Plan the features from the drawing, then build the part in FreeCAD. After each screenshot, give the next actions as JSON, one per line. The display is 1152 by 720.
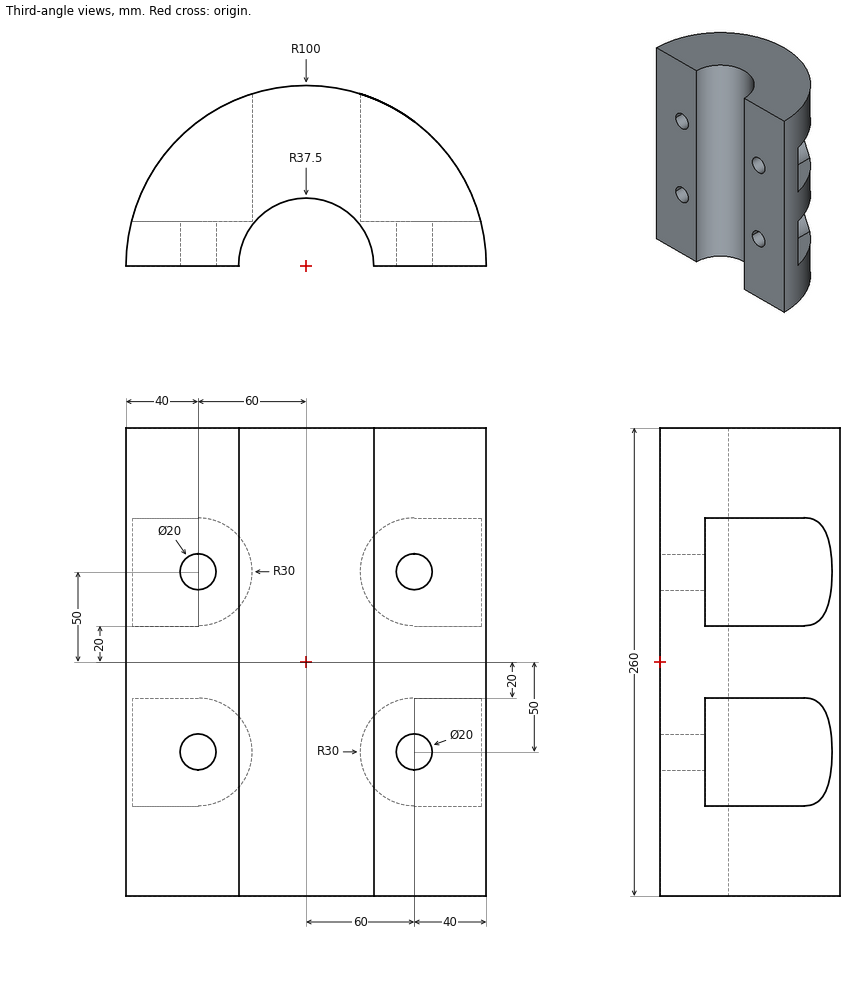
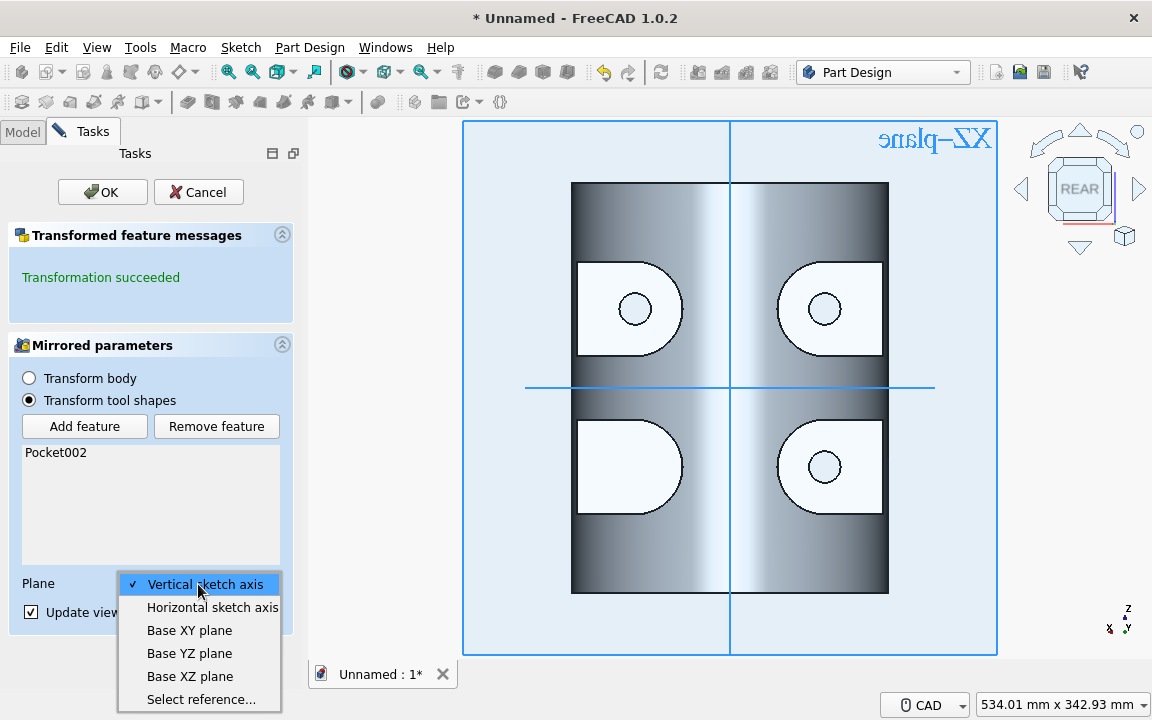
{"action": "left_click", "coordinate": [198, 654]}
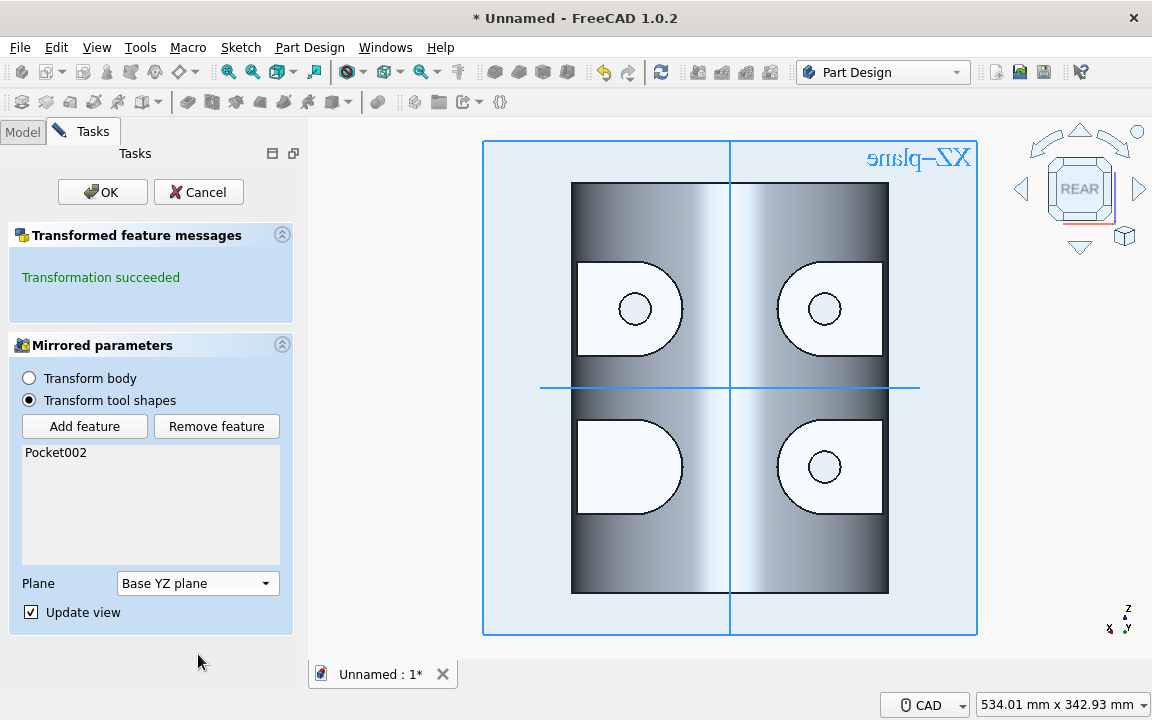
{"action": "left_click", "coordinate": [103, 192]}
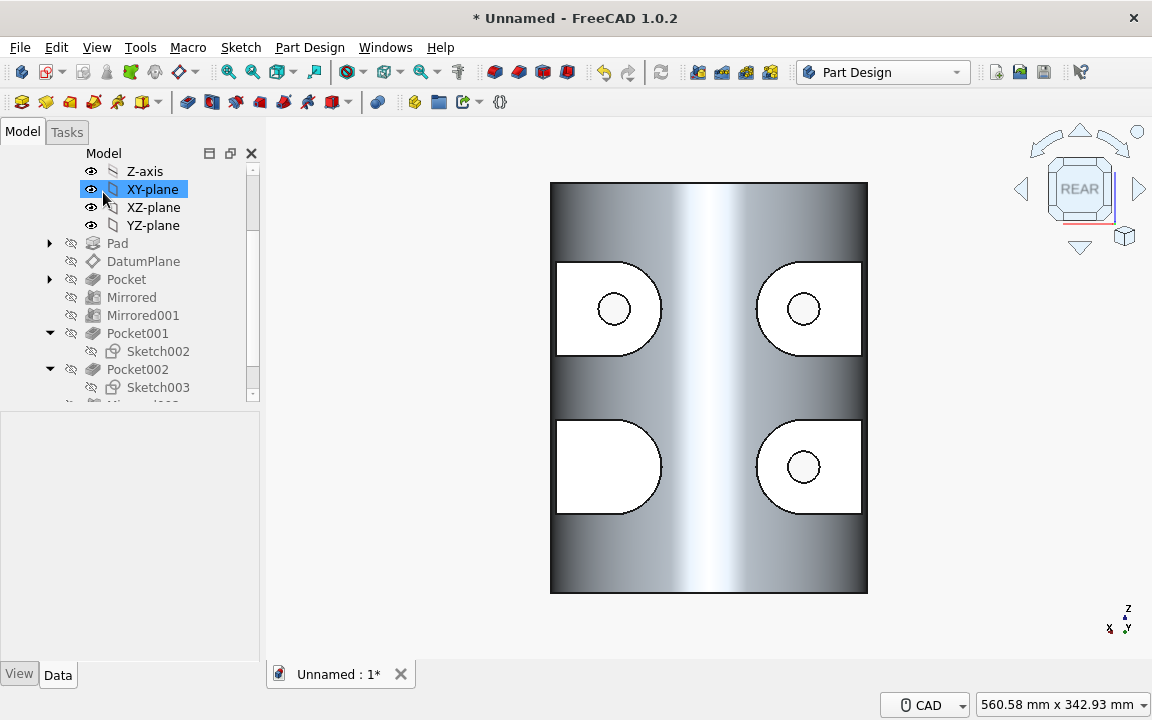
{"action": "left_click", "coordinate": [609, 466]}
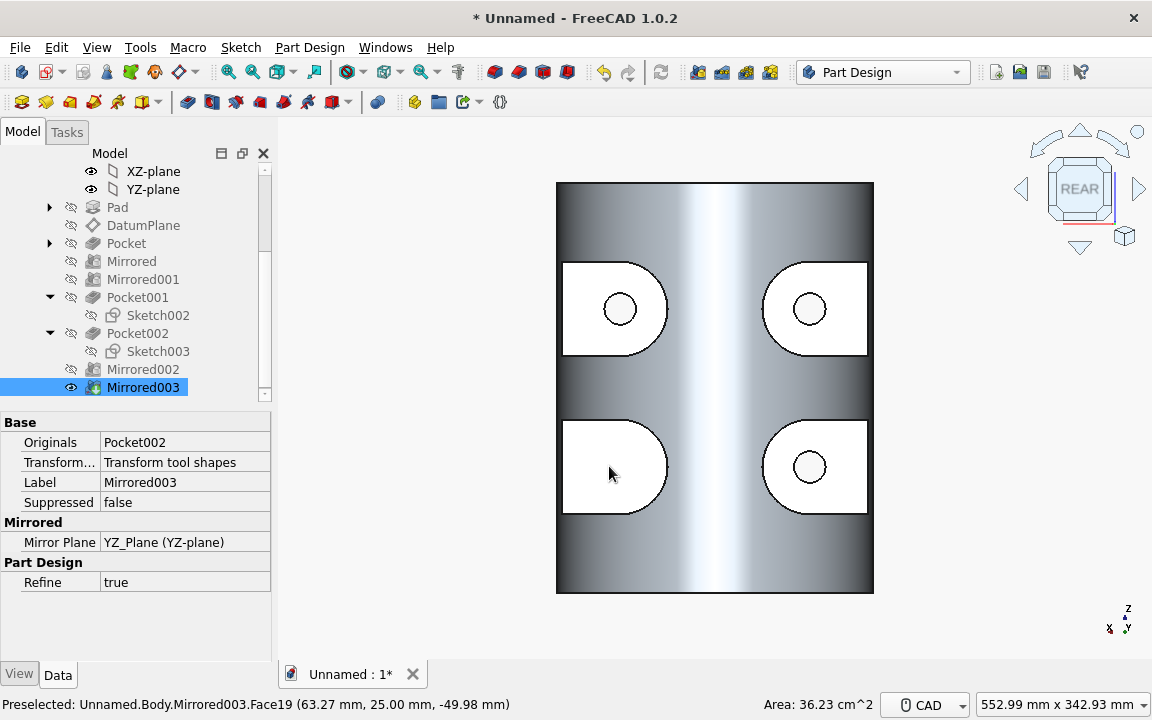
{"action": "left_click", "coordinate": [46, 72]}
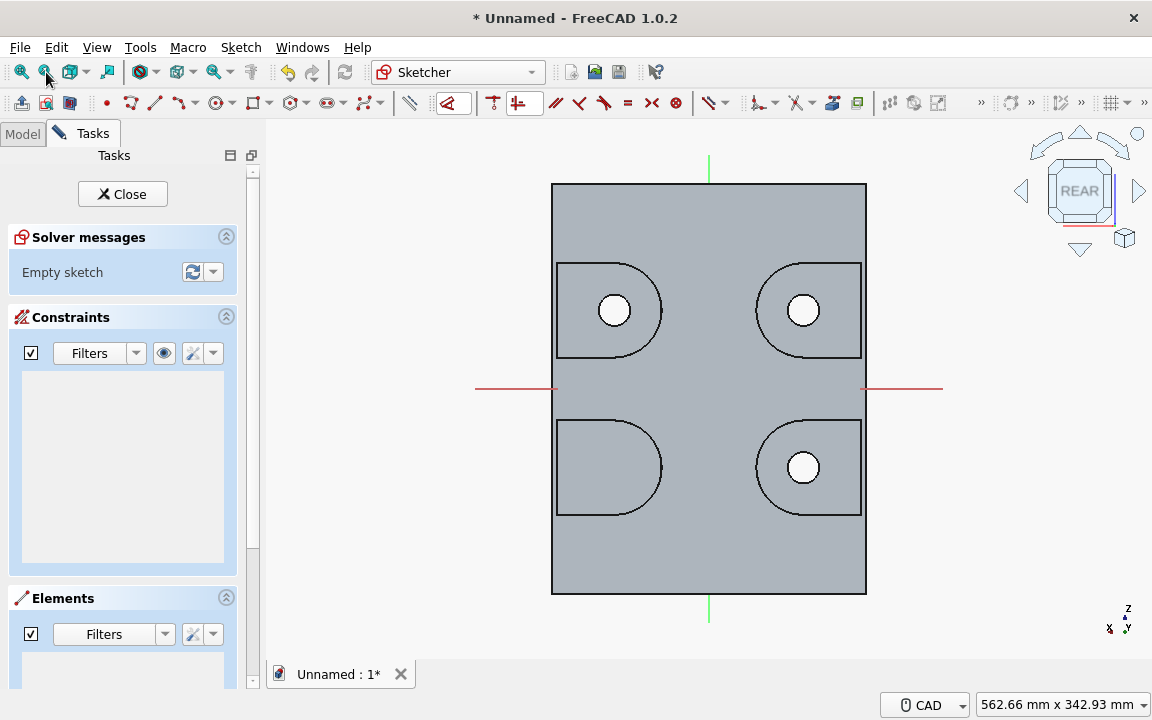
{"action": "key", "text": "q s"}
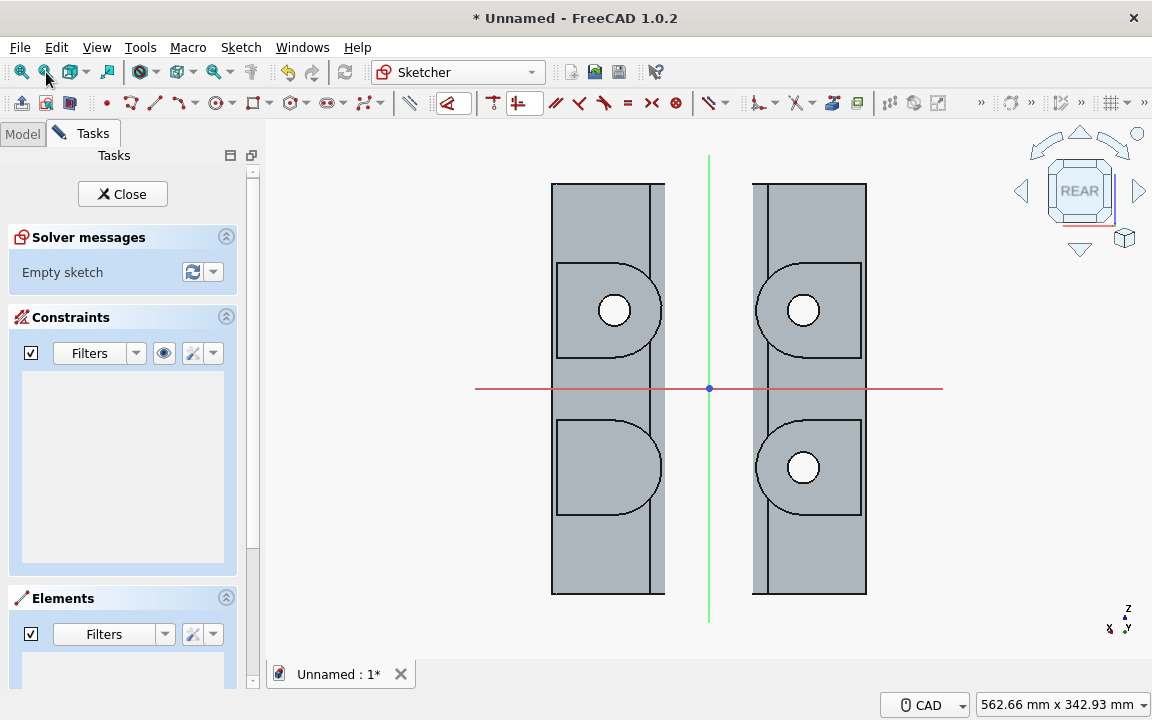
{"action": "scroll", "coordinate": [612, 476], "scroll_direction": "up", "scroll_amount": 12}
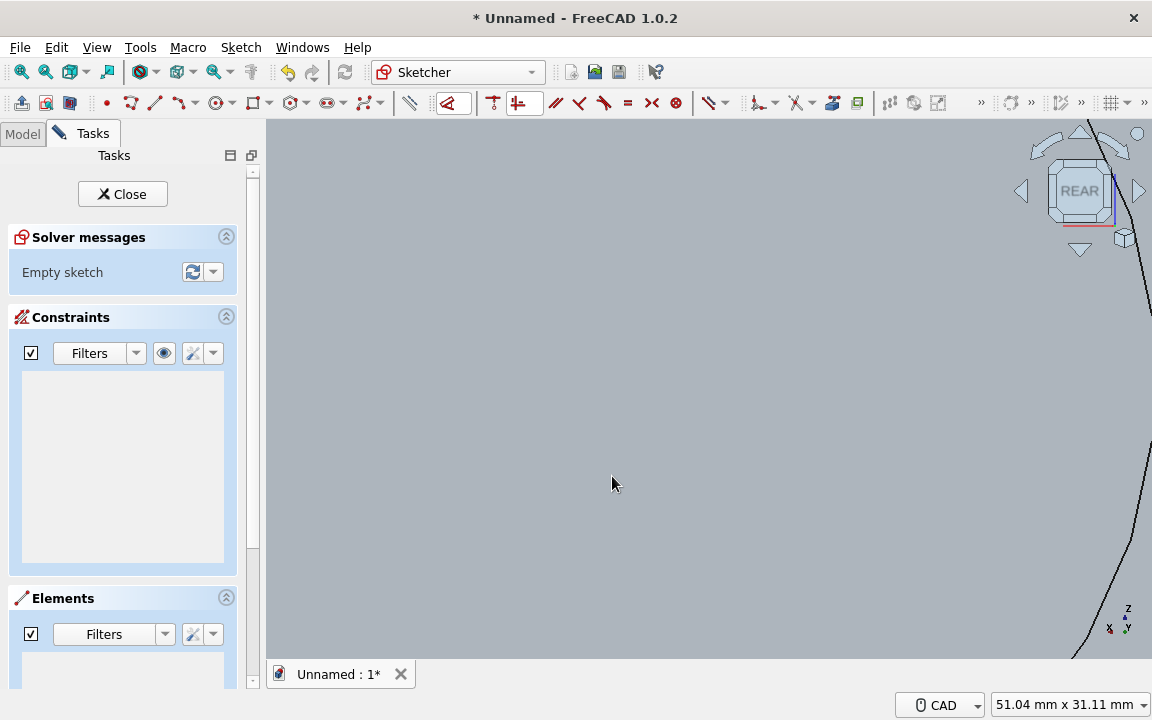
{"action": "key", "text": "g c"}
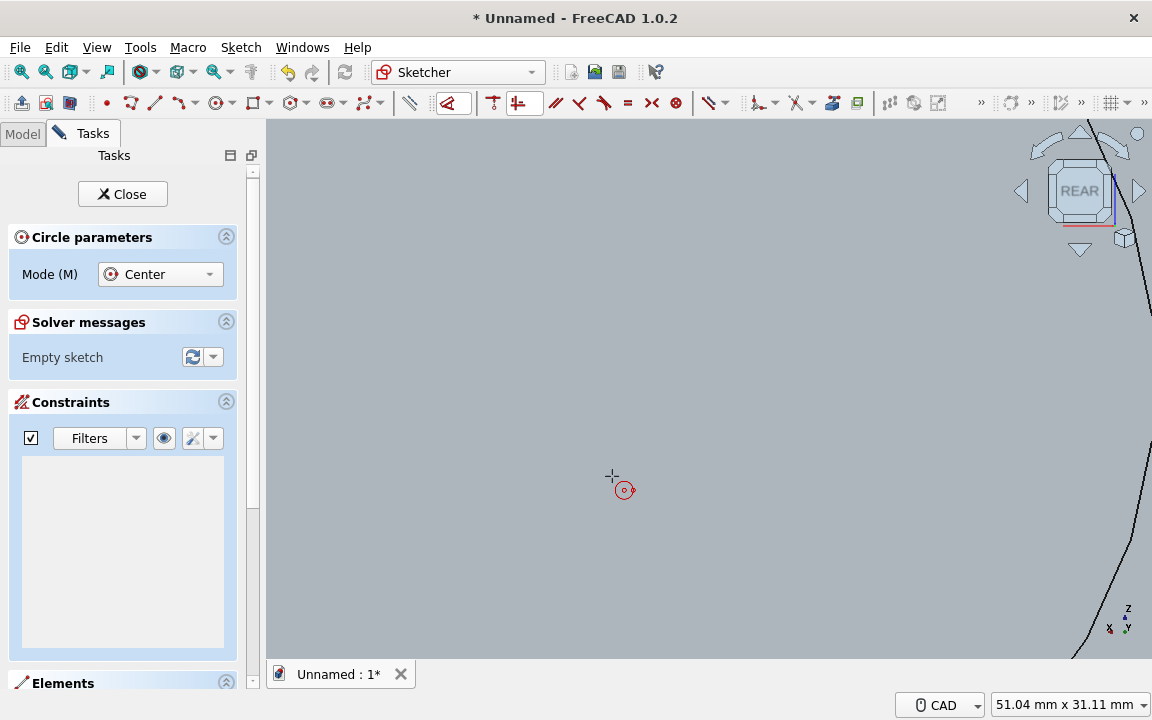
{"action": "left_click", "coordinate": [636, 378]}
{"action": "left_click", "coordinate": [759, 256]}
{"action": "key", "text": "Escape"}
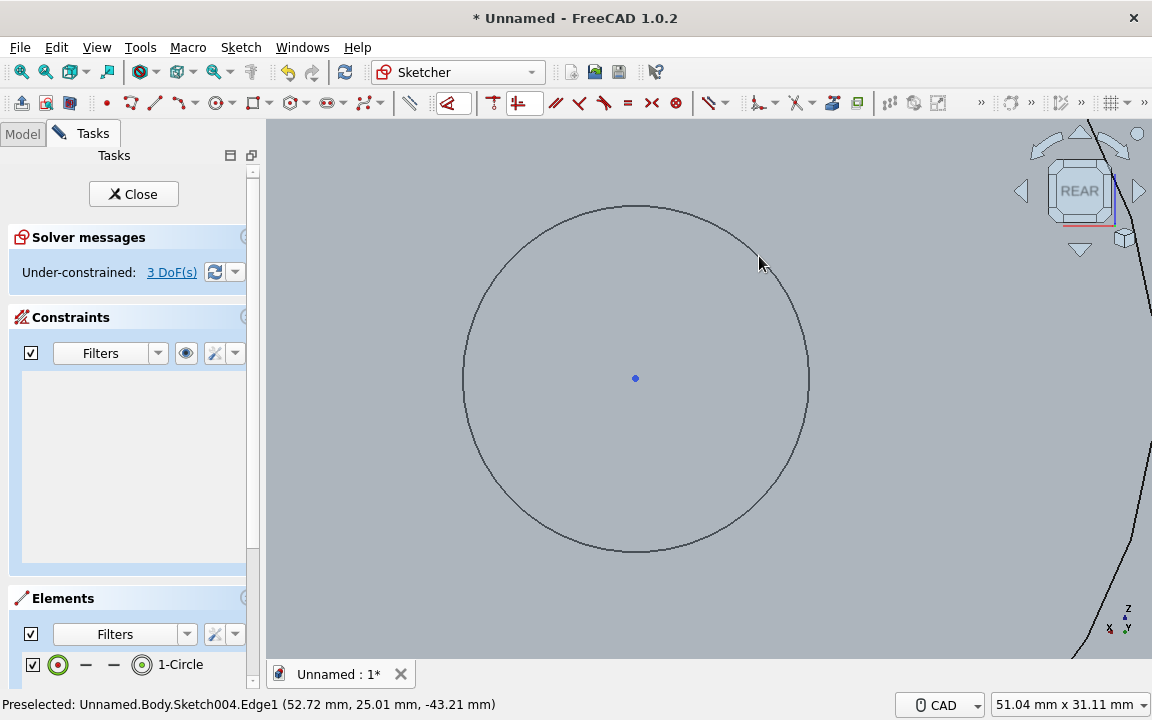
{"action": "left_click", "coordinate": [758, 256]}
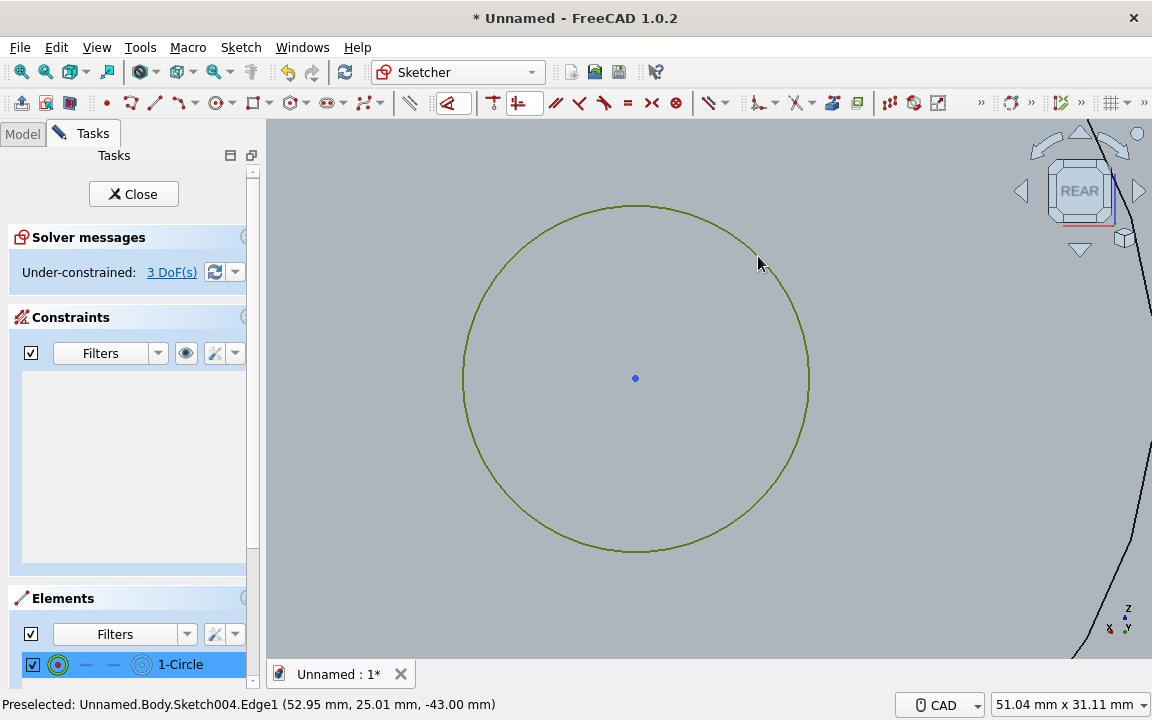
{"action": "key", "text": "k o"}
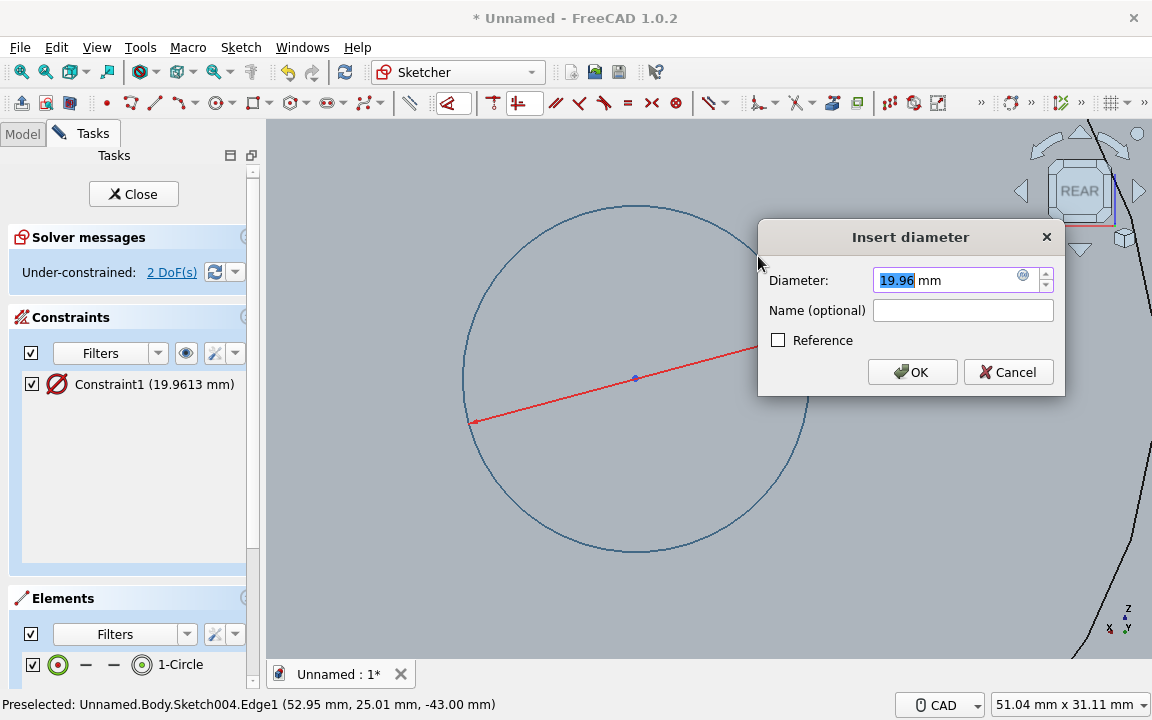
{"action": "type", "text": "20"}
{"action": "key", "text": "Return"}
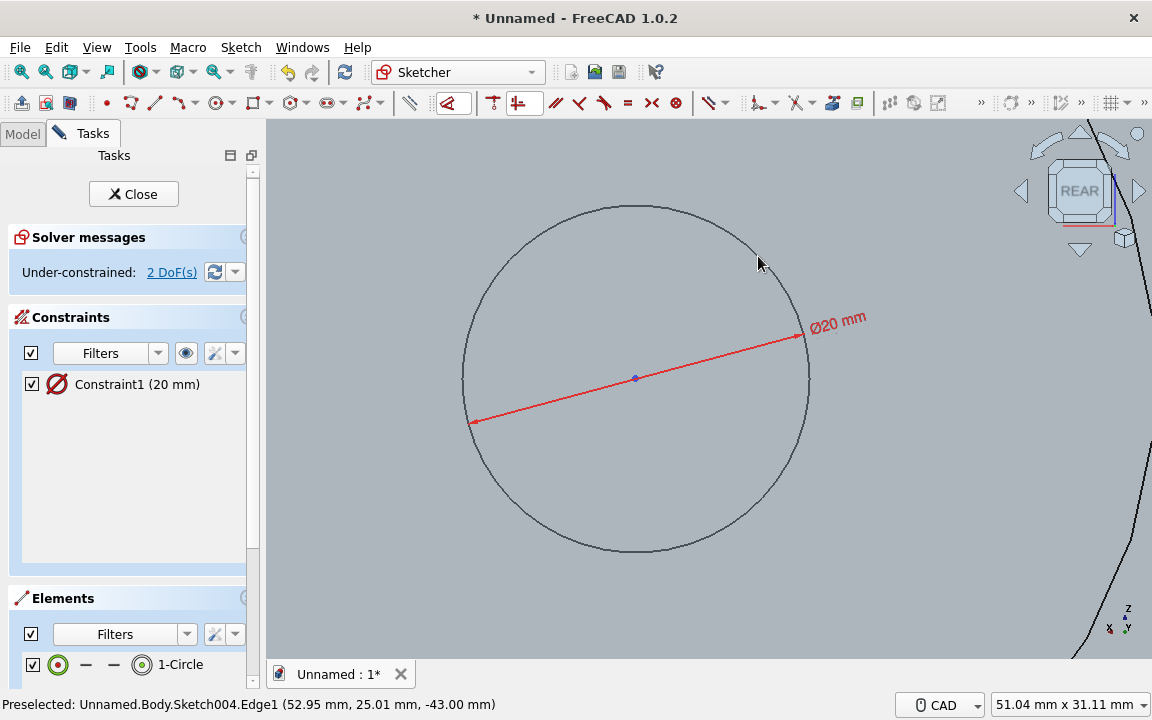
{"action": "left_click", "coordinate": [636, 379]}